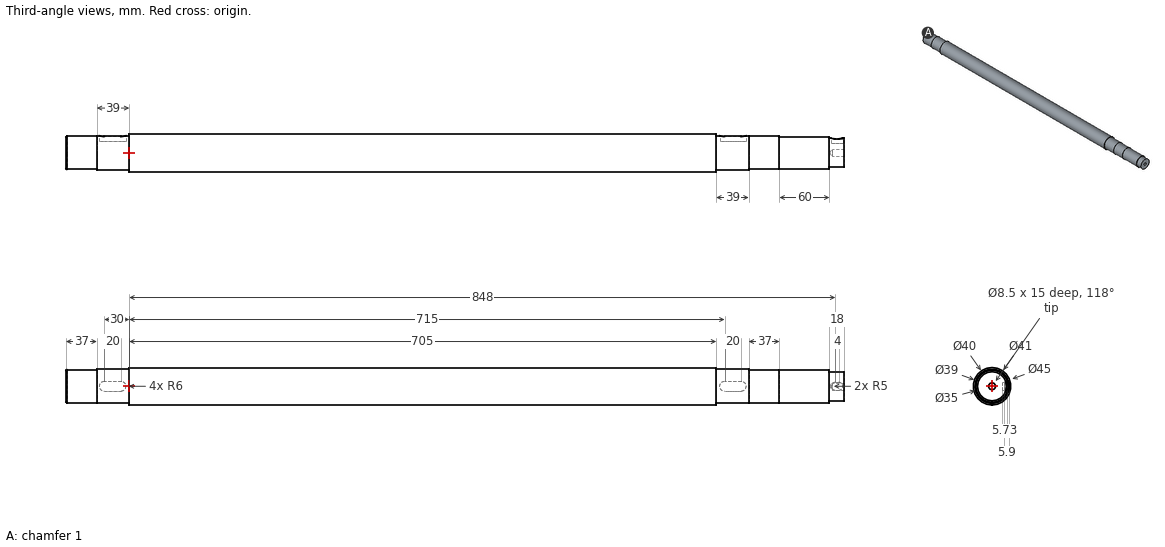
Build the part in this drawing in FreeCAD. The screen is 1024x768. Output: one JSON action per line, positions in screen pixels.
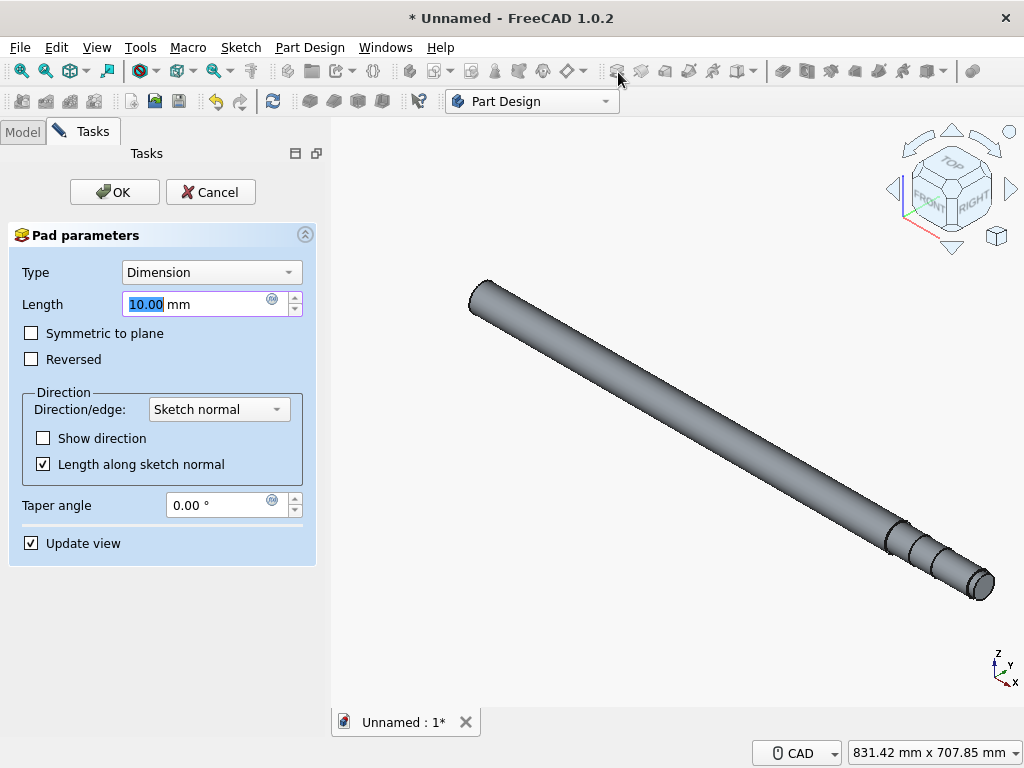
{"action": "type", "text": "18"}
{"action": "key", "text": "Tab"}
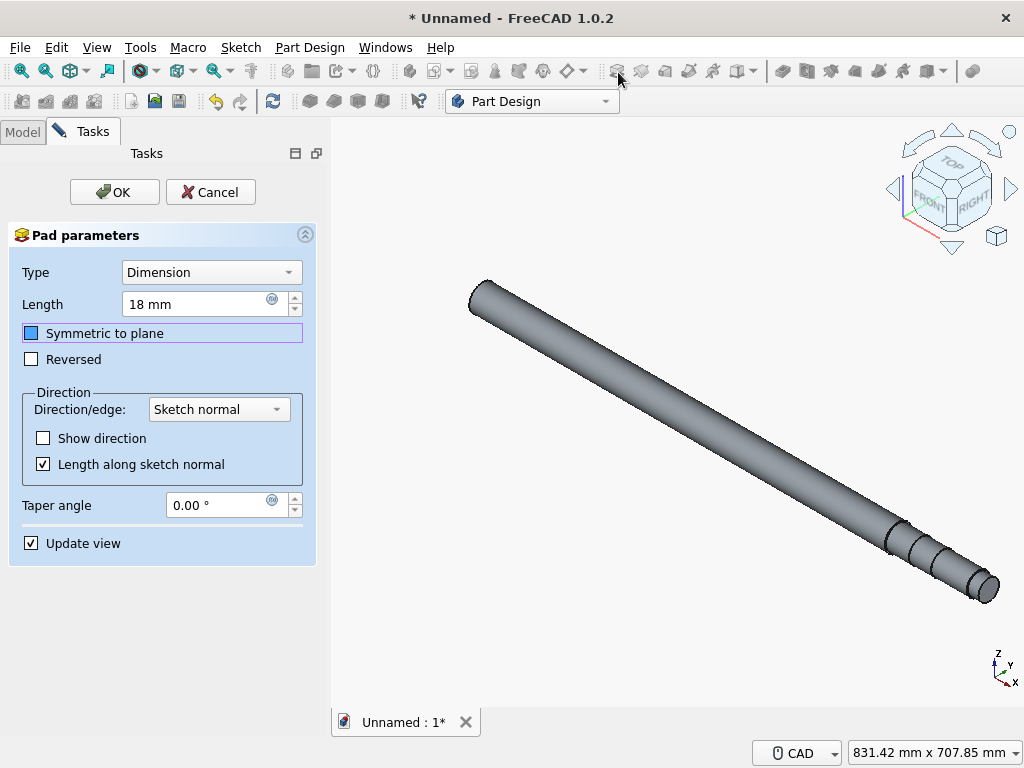
{"action": "left_click", "coordinate": [115, 192]}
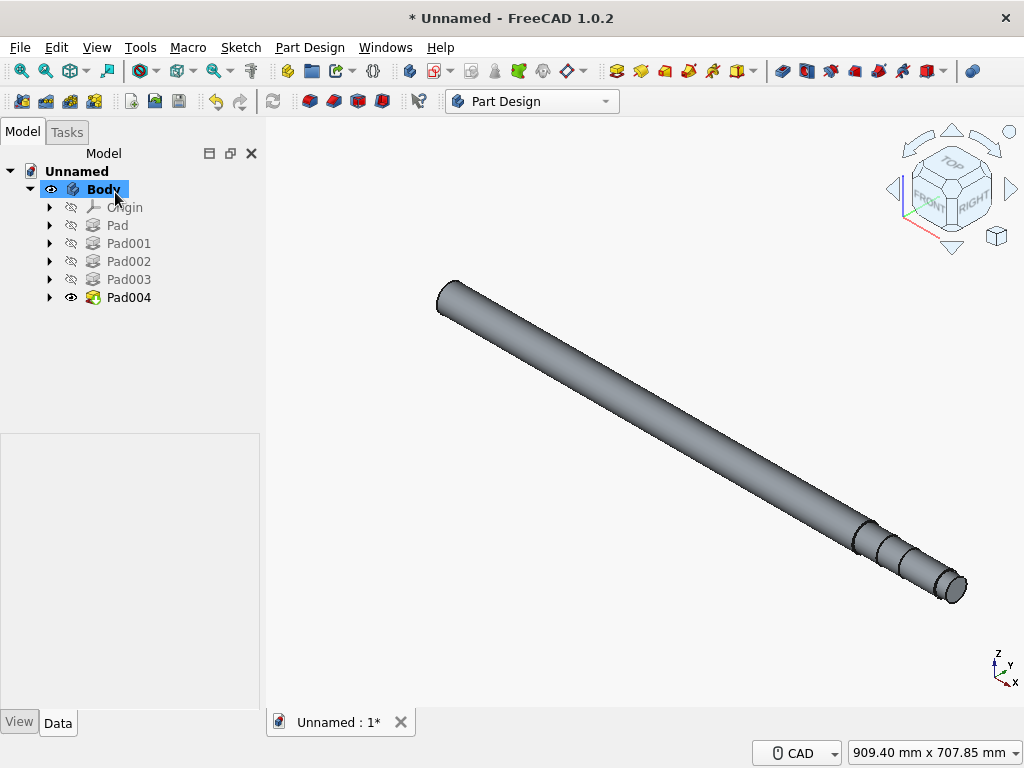
{"action": "left_click", "coordinate": [50, 207]}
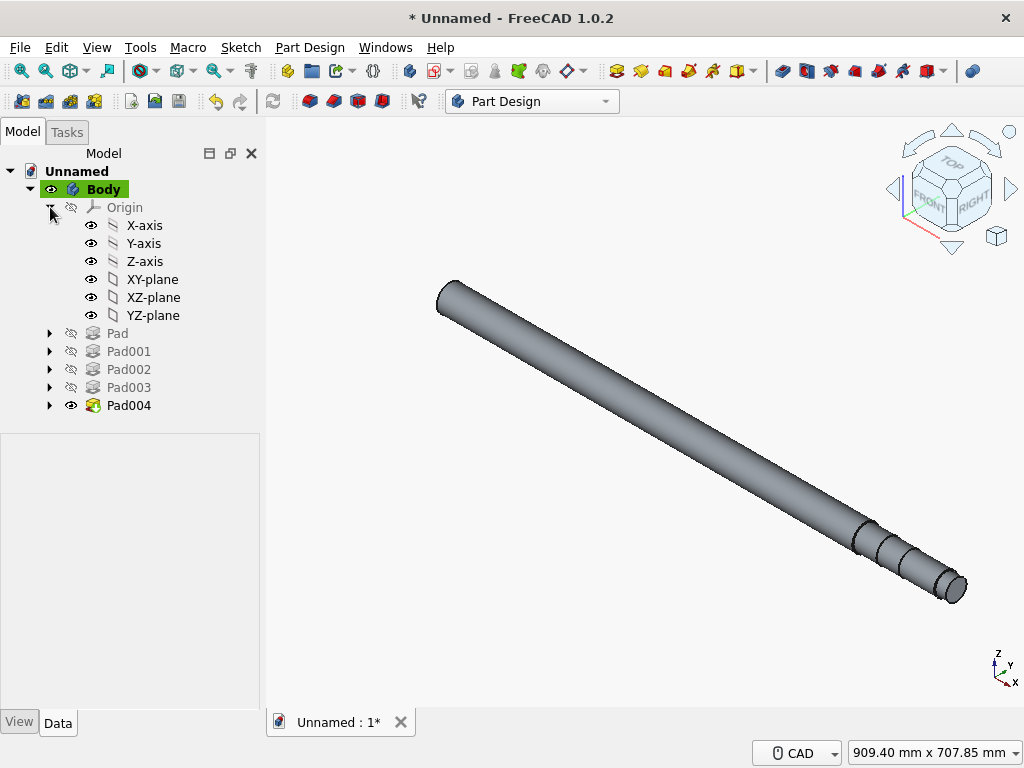
{"action": "left_click", "coordinate": [136, 315]}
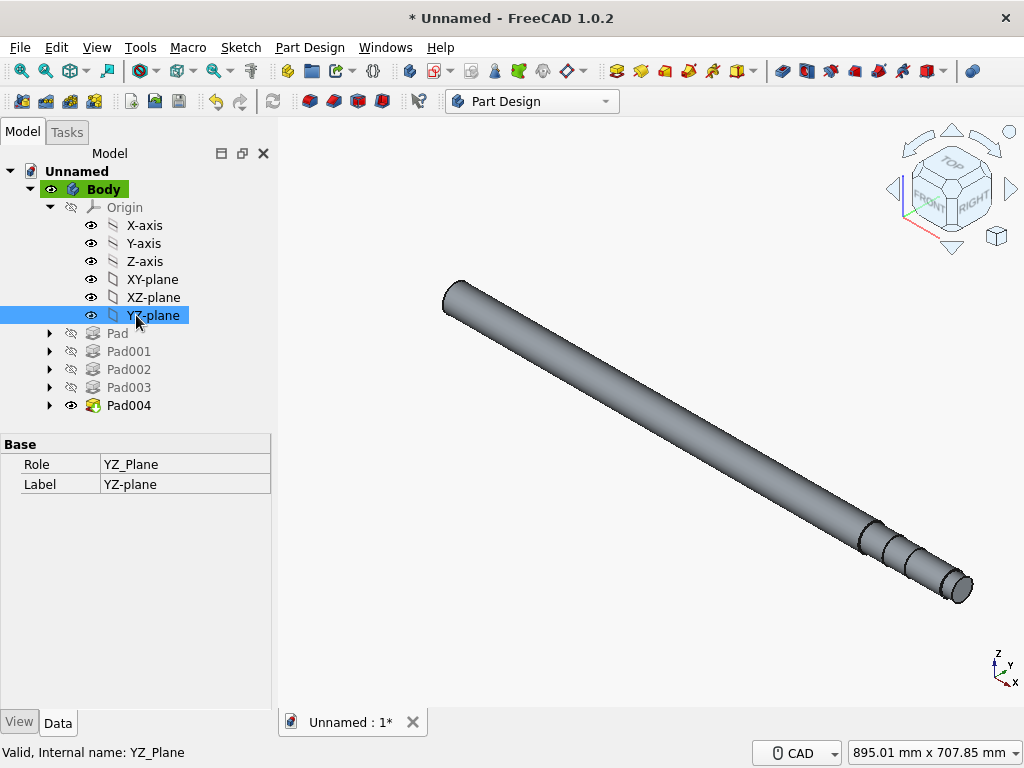
{"action": "left_click", "coordinate": [568, 72]}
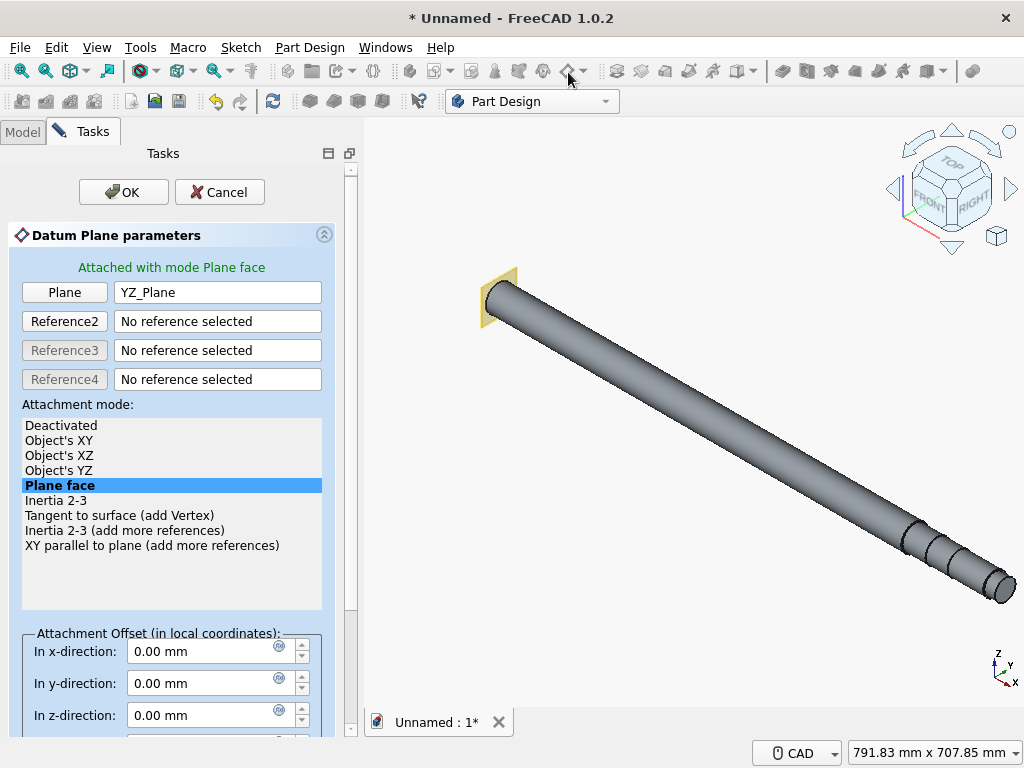
{"action": "triple_click", "coordinate": [210, 715]}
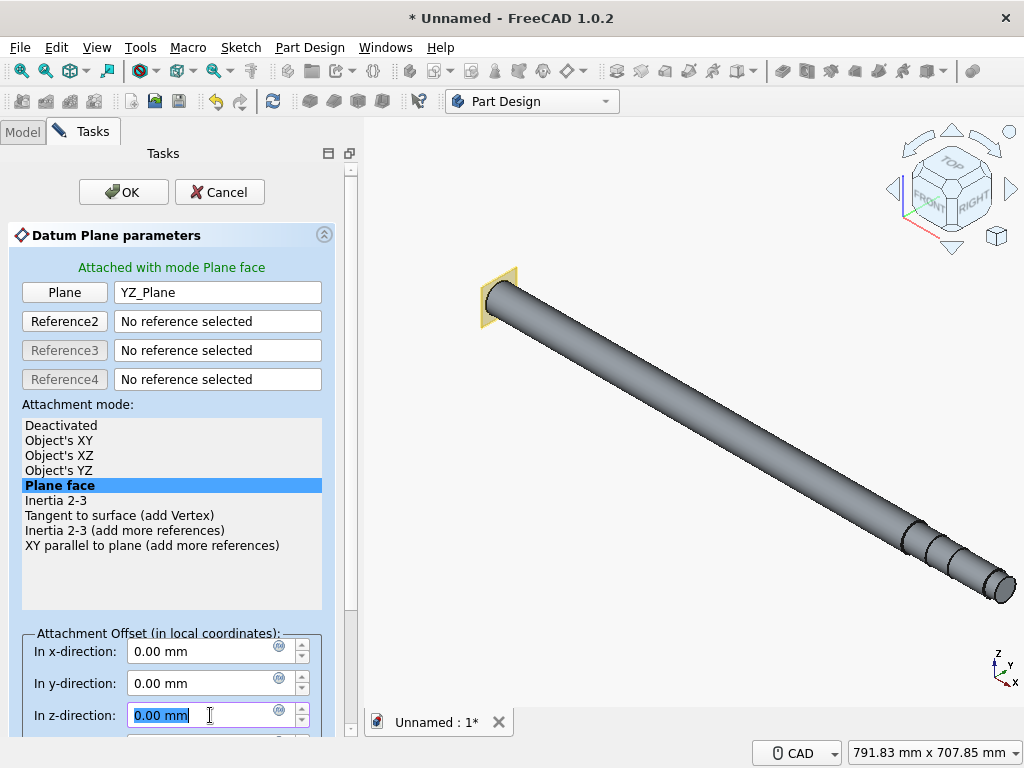
{"action": "type", "text": "-39"}
{"action": "key", "text": "Tab"}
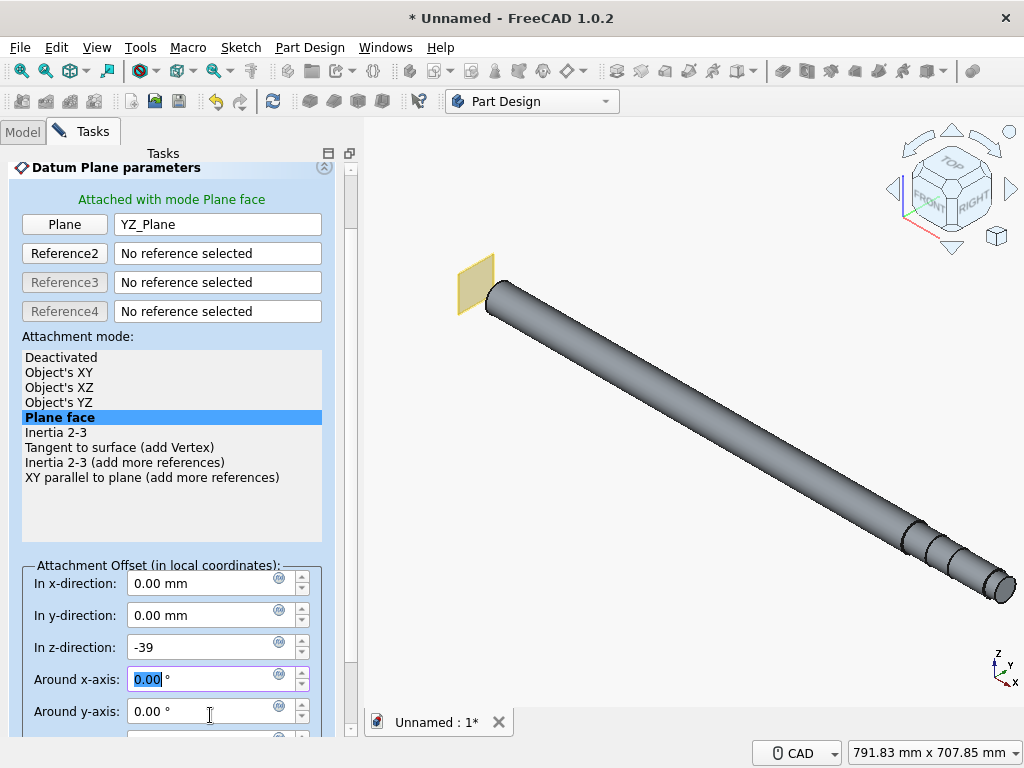
{"action": "scroll", "coordinate": [351, 450], "scroll_direction": "up", "scroll_amount": 2}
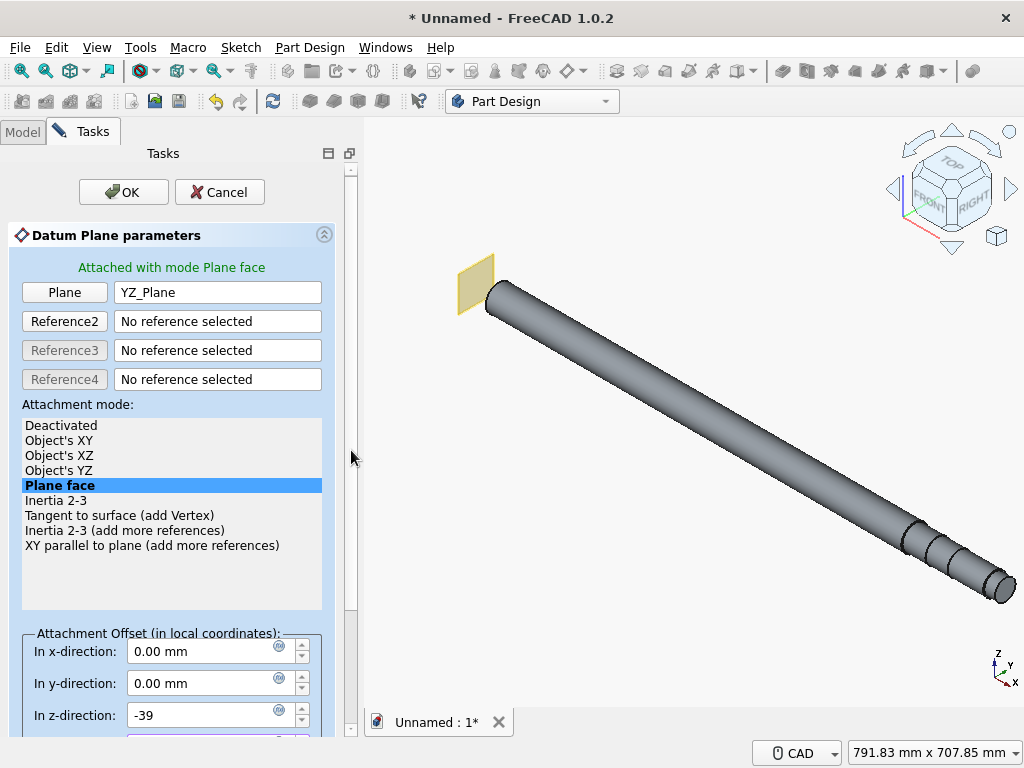
{"action": "left_click", "coordinate": [124, 192]}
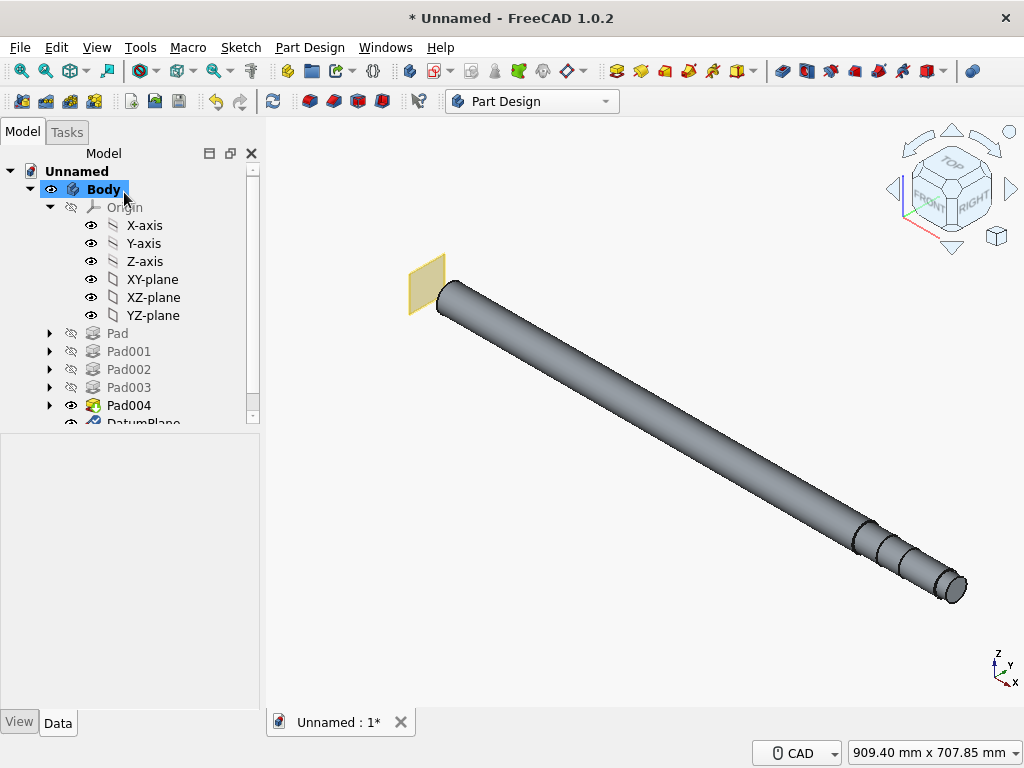
{"action": "left_click", "coordinate": [116, 423]}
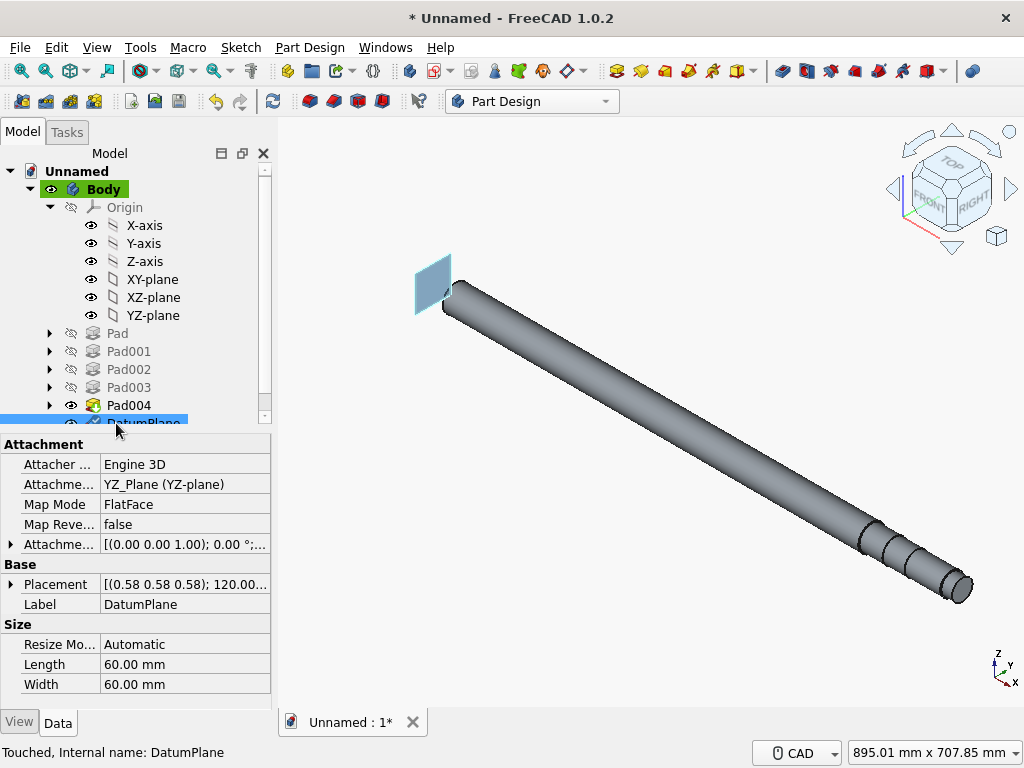
{"action": "left_click", "coordinate": [434, 72]}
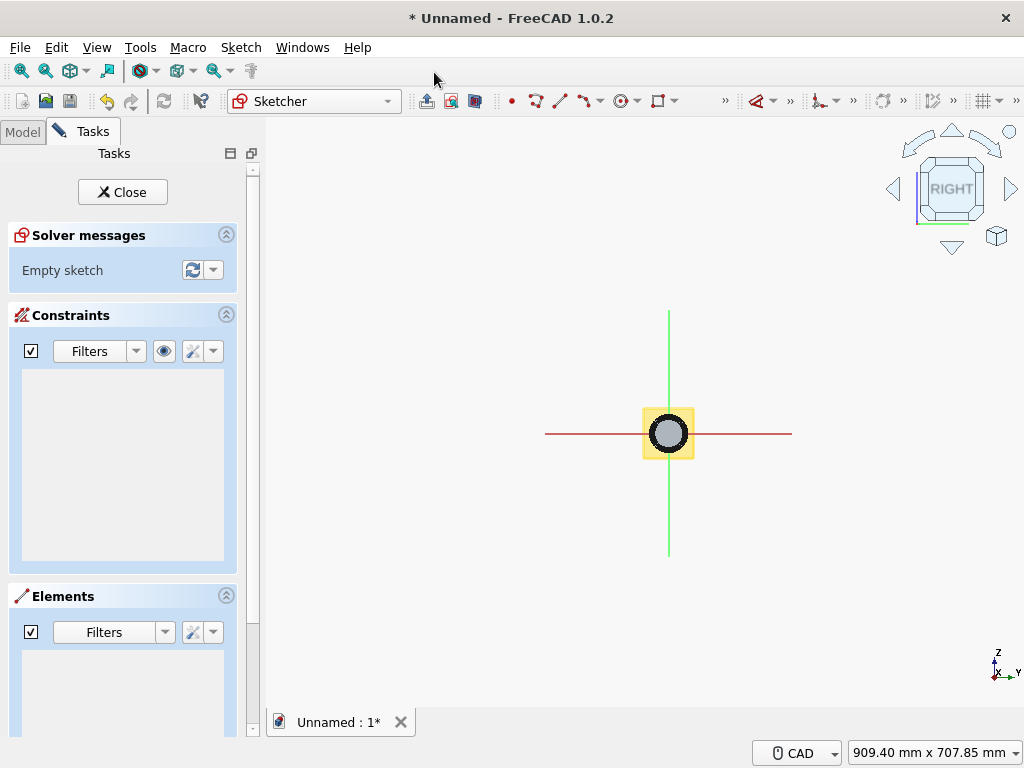
{"action": "left_click", "coordinate": [476, 102]}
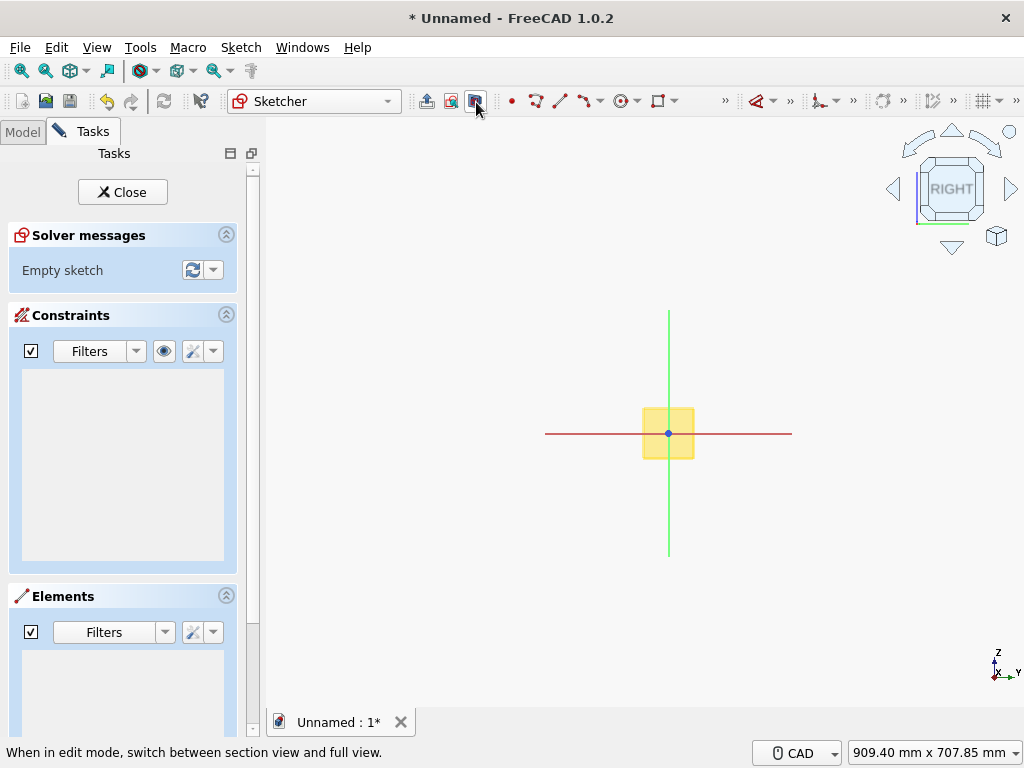
{"action": "scroll", "coordinate": [678, 436], "scroll_direction": "up", "scroll_amount": 12}